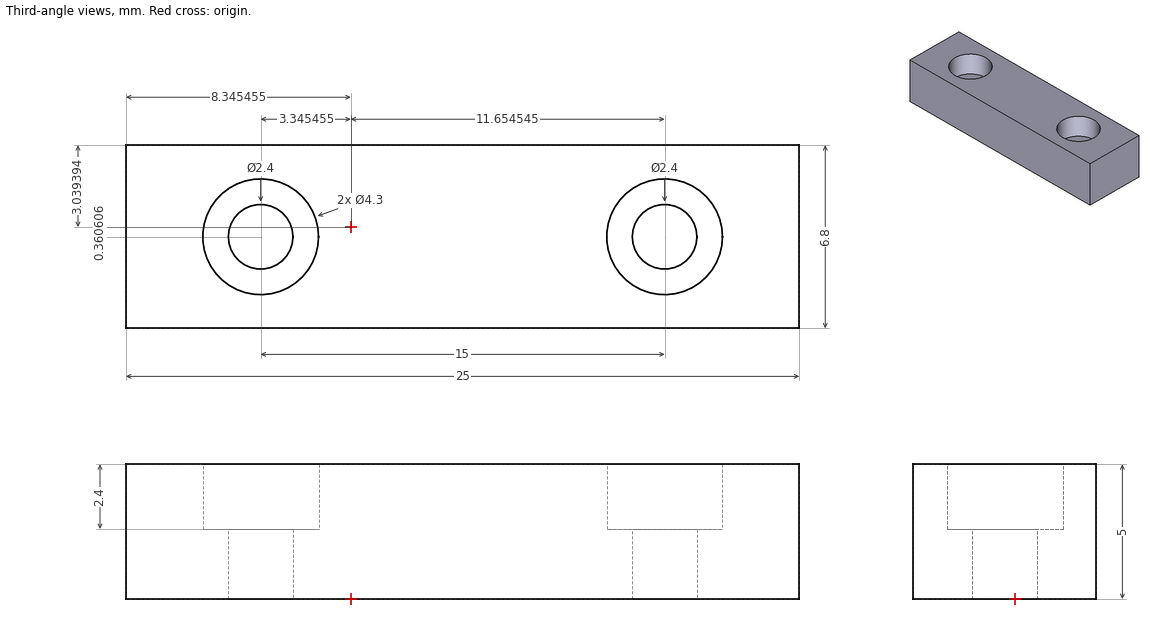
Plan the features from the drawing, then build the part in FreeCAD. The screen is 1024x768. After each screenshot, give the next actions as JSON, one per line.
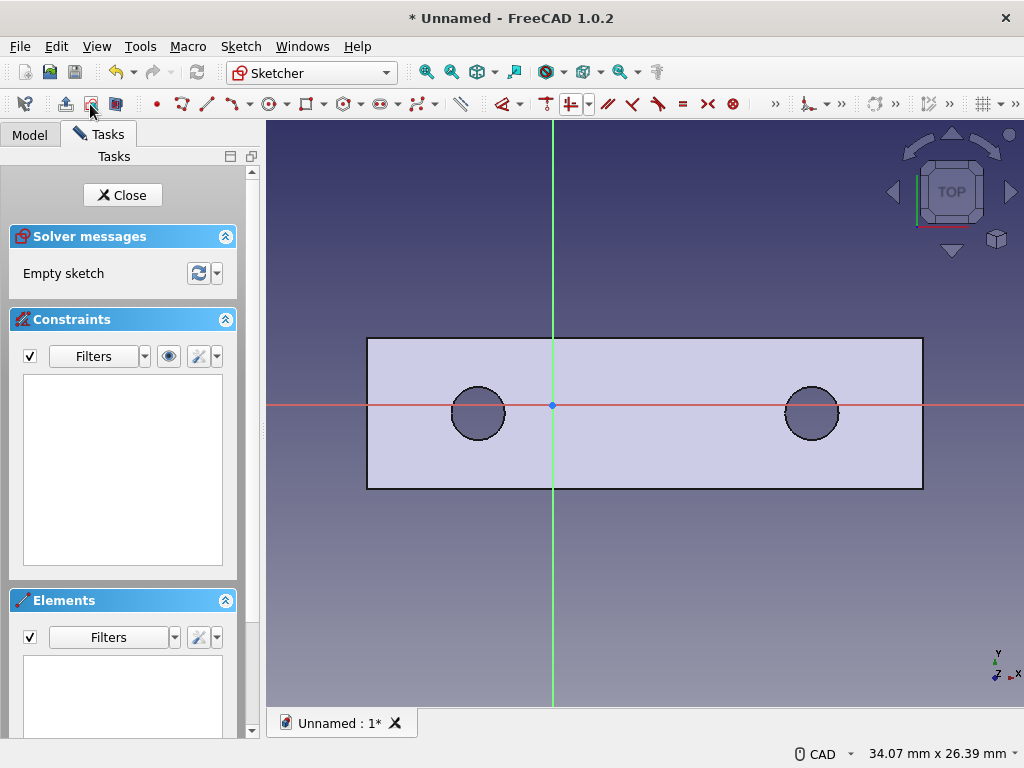
{"action": "scroll", "coordinate": [294, 414], "scroll_direction": "down", "scroll_amount": 1}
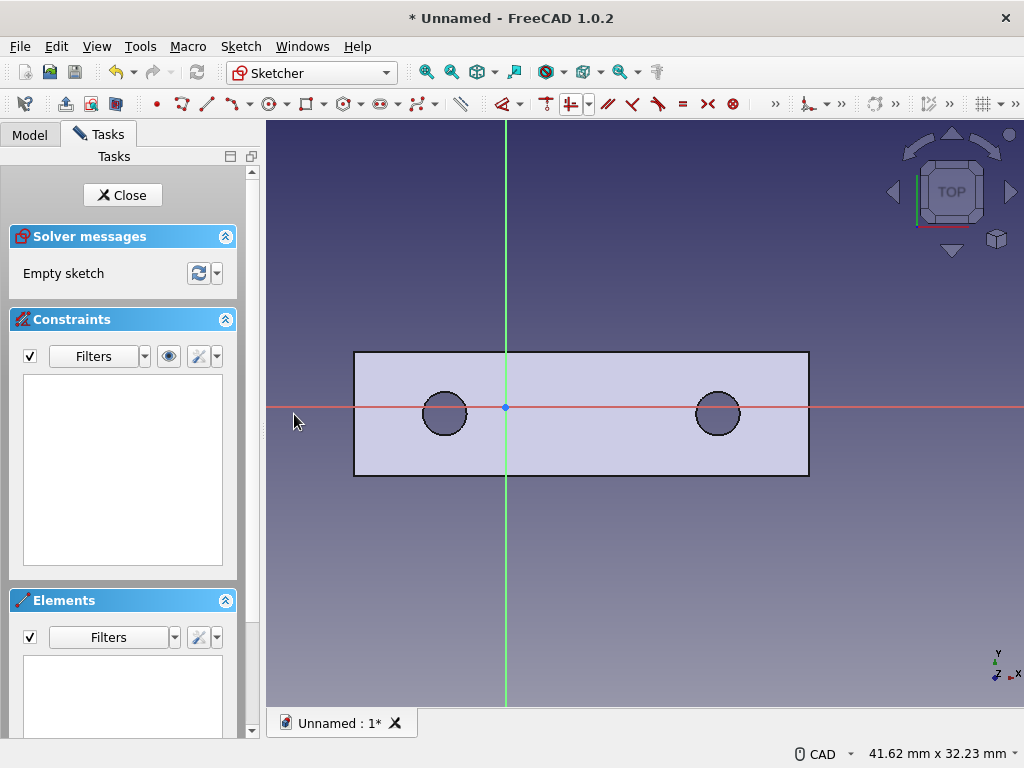
{"action": "key", "text": "g c"}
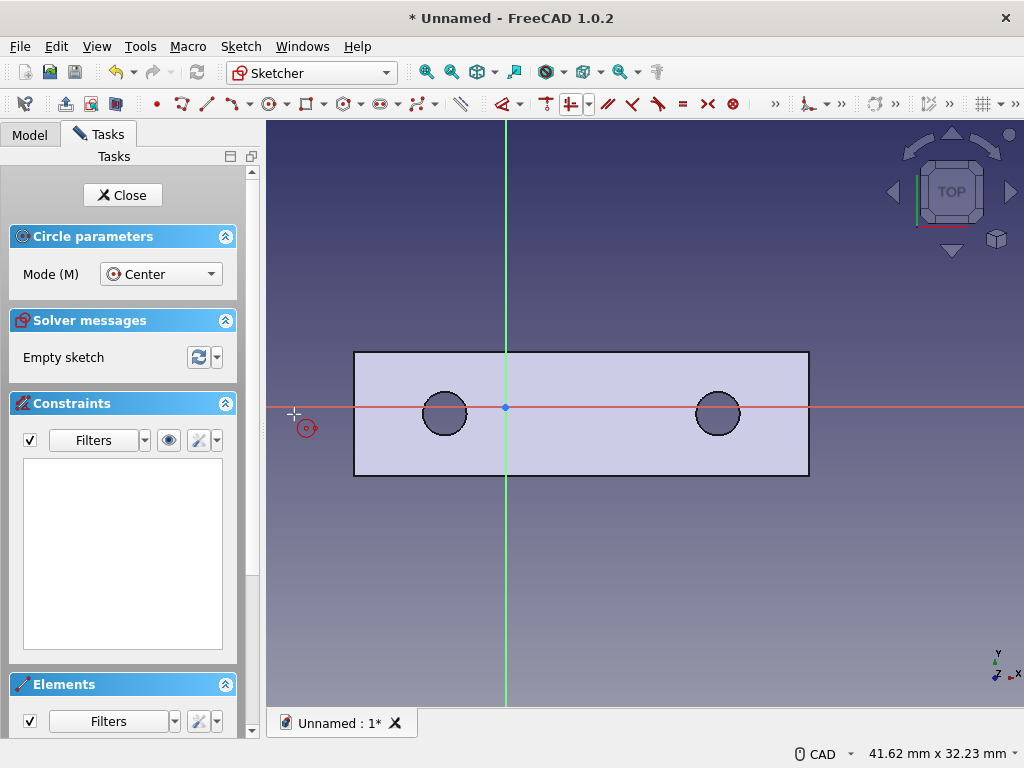
{"action": "scroll", "coordinate": [445, 414], "scroll_direction": "up", "scroll_amount": 5}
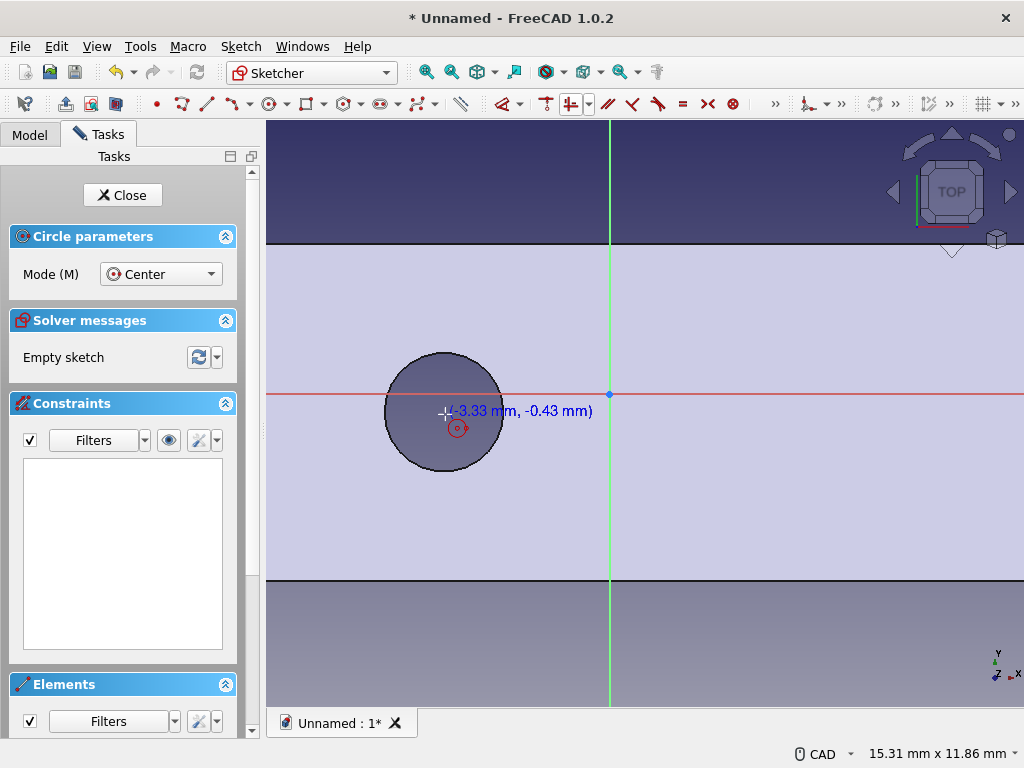
{"action": "left_click", "coordinate": [444, 412]}
{"action": "mouse_move", "coordinate": [519, 337]}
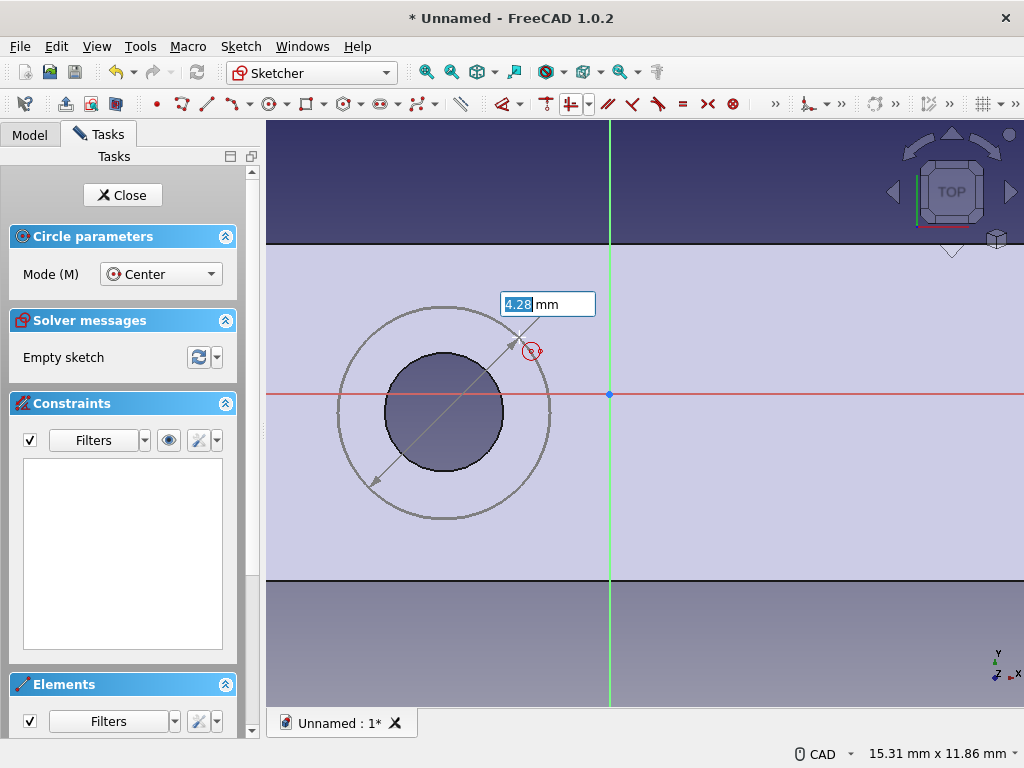
{"action": "type", "text": "4.3"}
{"action": "key", "text": "Return"}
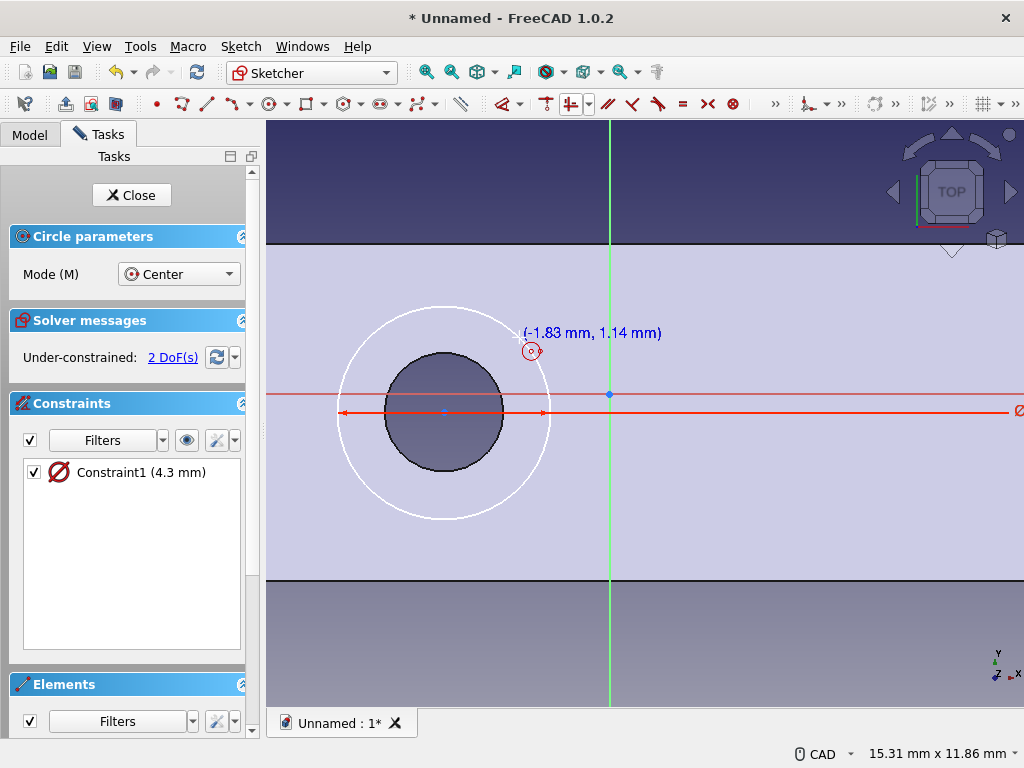
{"action": "scroll", "coordinate": [382, 415], "scroll_direction": "down", "scroll_amount": 4}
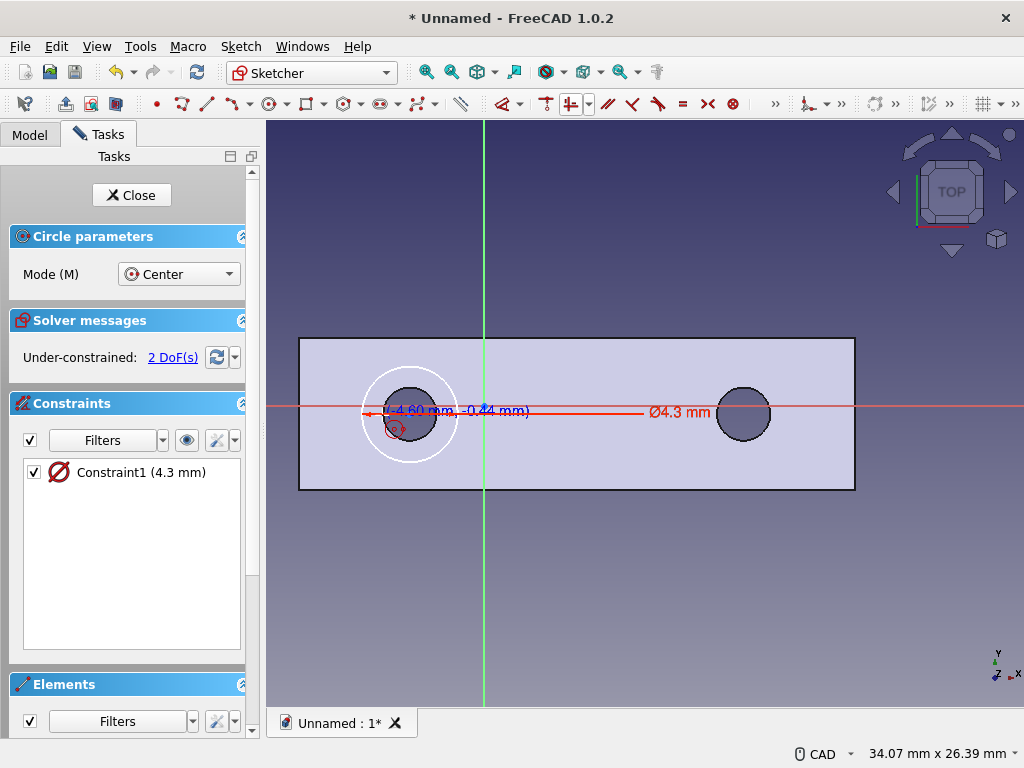
{"action": "scroll", "coordinate": [744, 414], "scroll_direction": "up", "scroll_amount": 4}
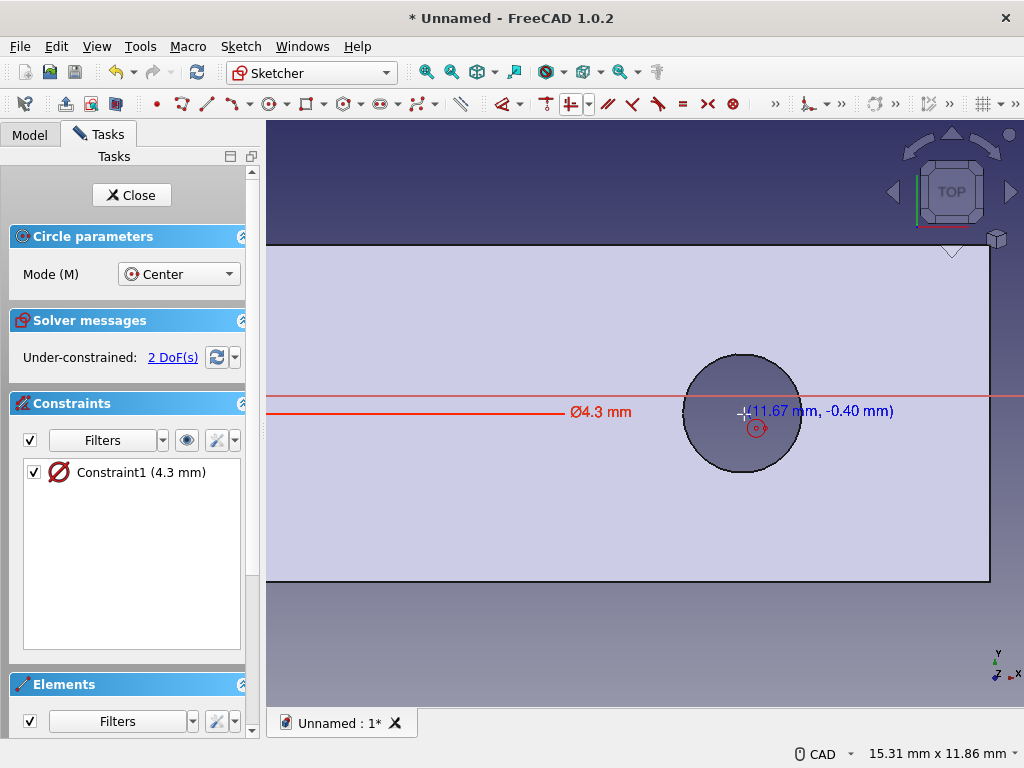
{"action": "left_click", "coordinate": [742, 413]}
{"action": "mouse_move", "coordinate": [818, 338]}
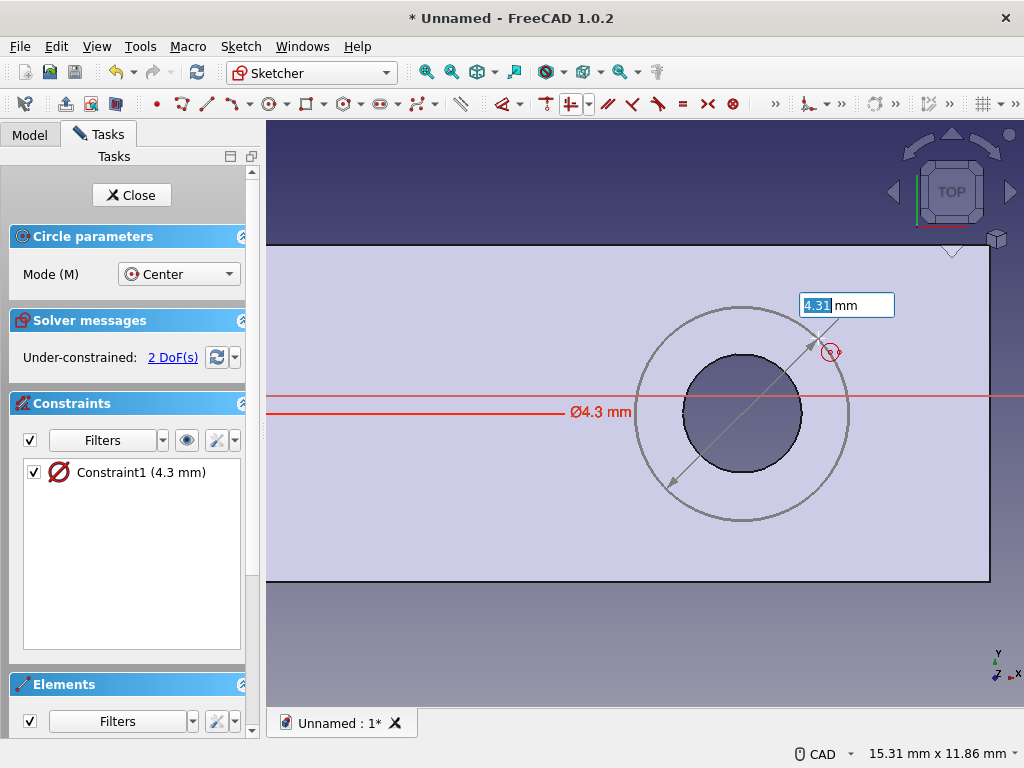
{"action": "type", "text": "4.3"}
{"action": "key", "text": "Return"}
{"action": "key", "text": "Escape"}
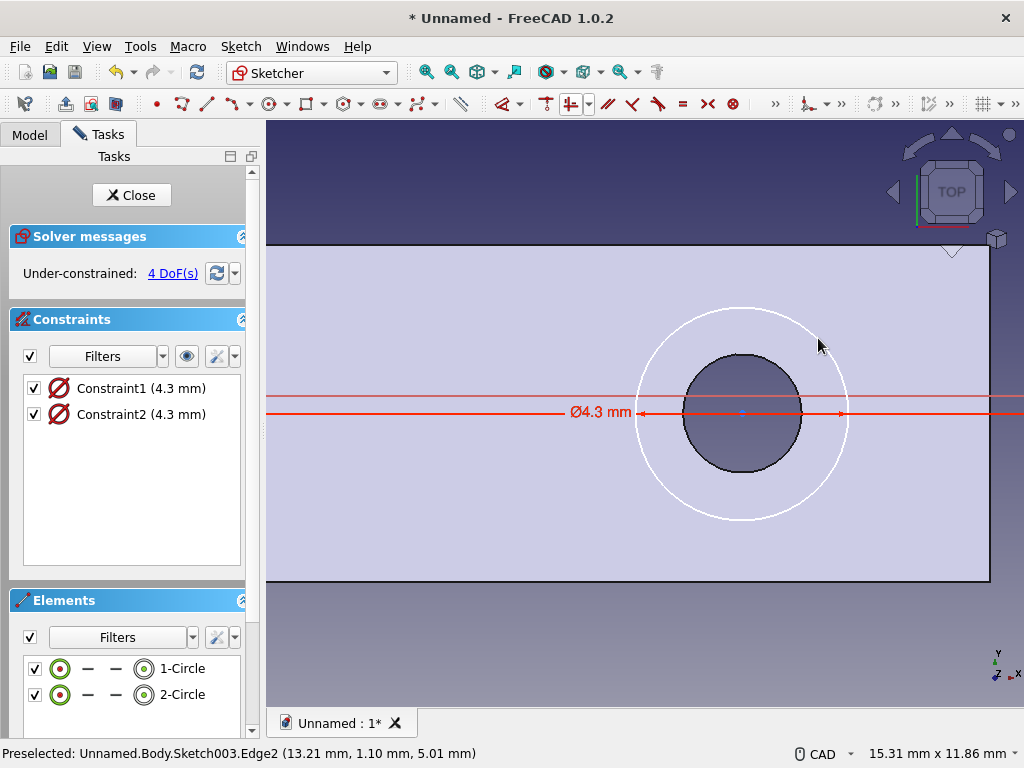
{"action": "key", "text": "d"}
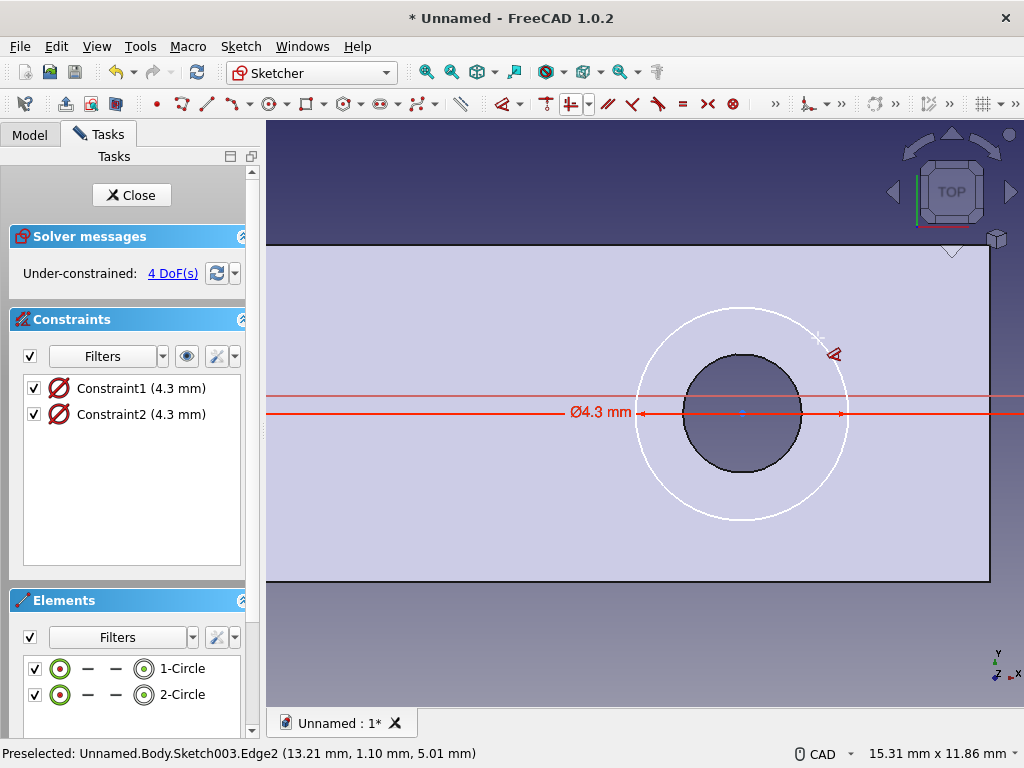
{"action": "scroll", "coordinate": [744, 414], "scroll_direction": "down", "scroll_amount": 4}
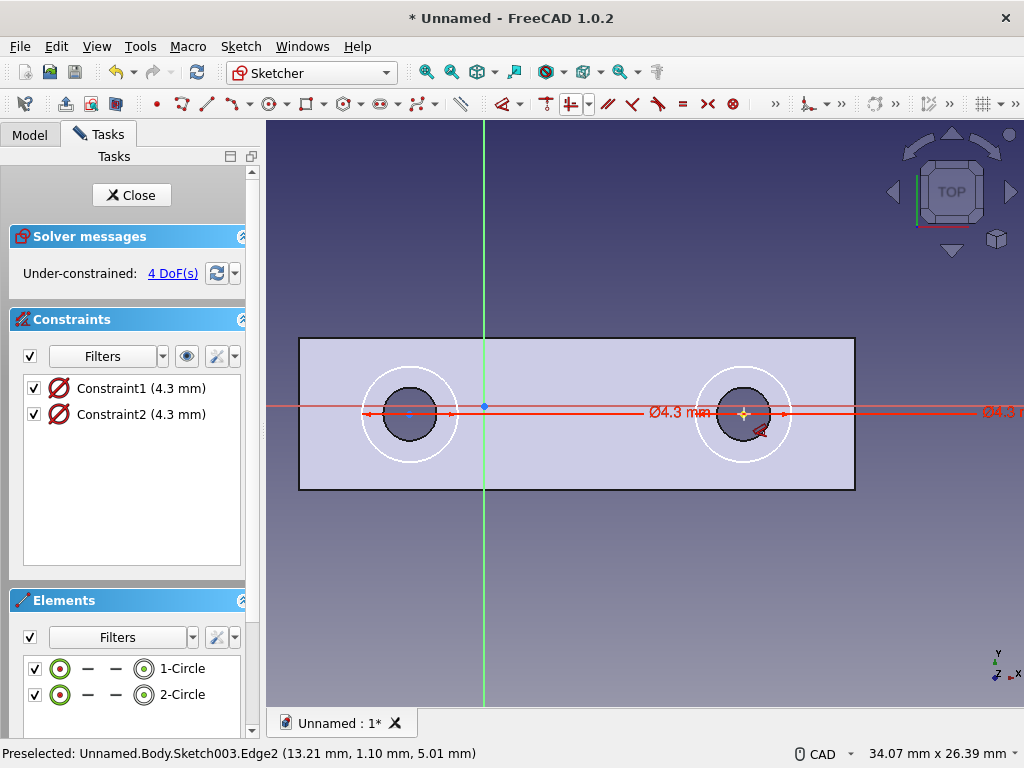
{"action": "left_click", "coordinate": [410, 414]}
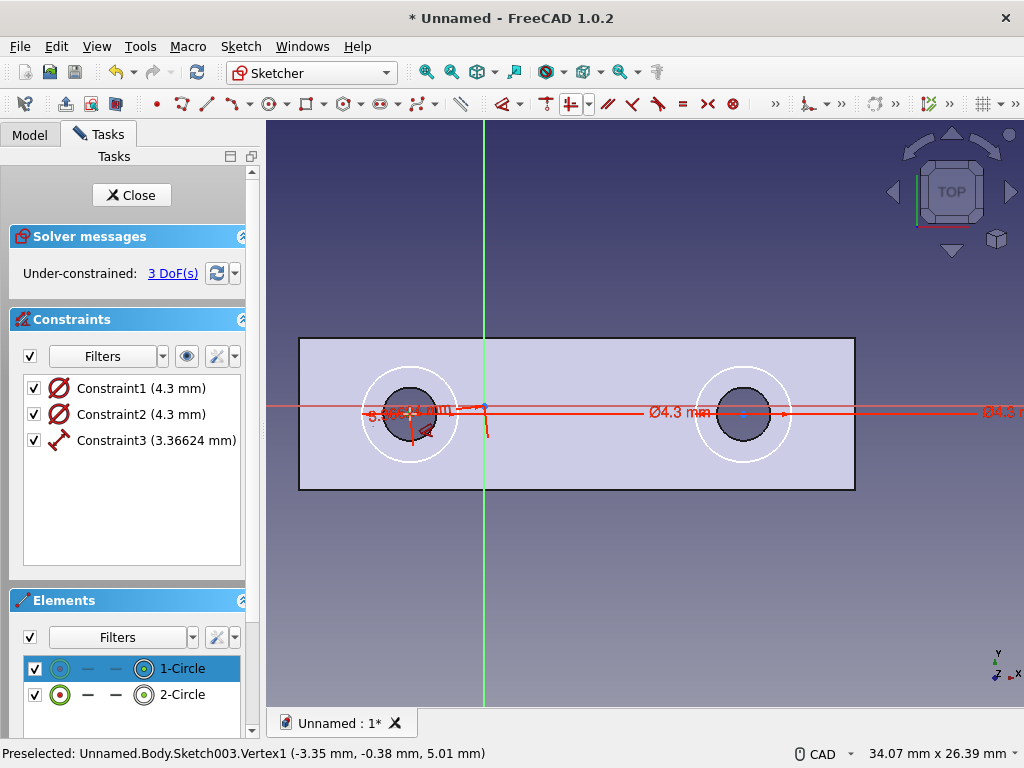
{"action": "left_click", "coordinate": [743, 414]}
{"action": "left_click", "coordinate": [577, 448]}